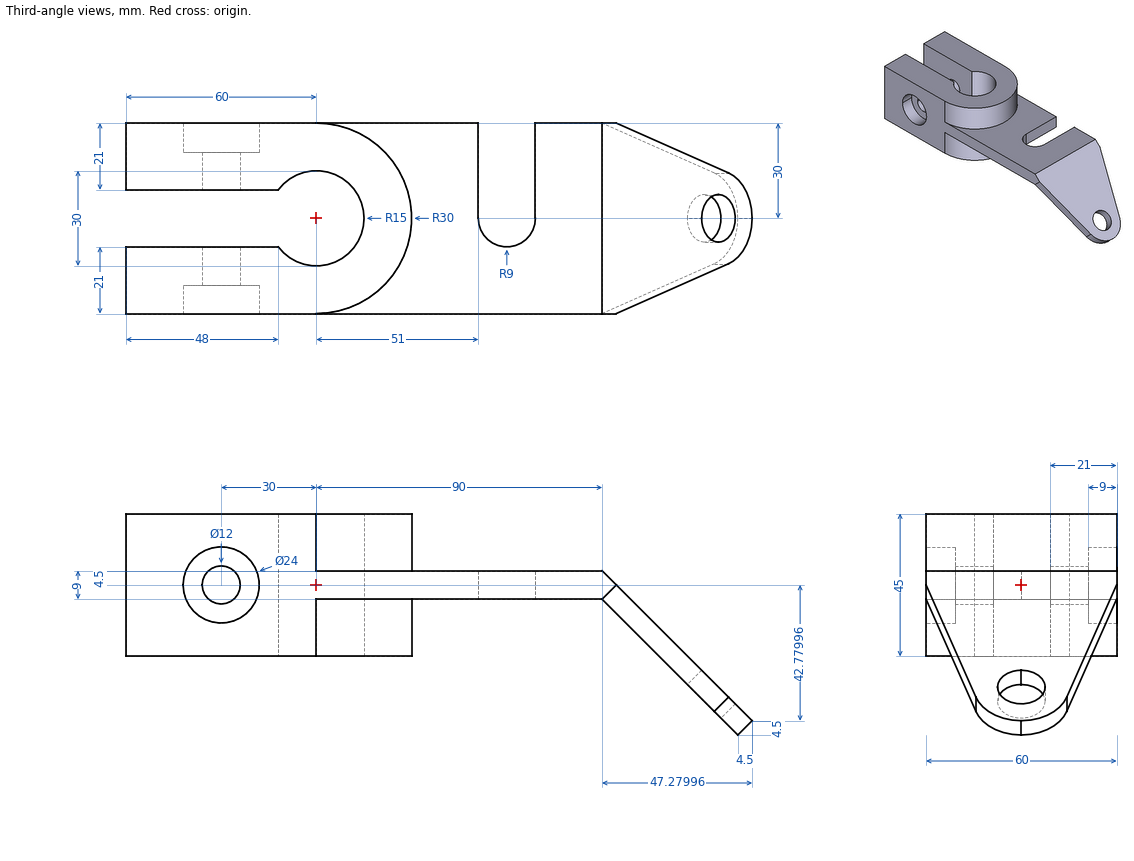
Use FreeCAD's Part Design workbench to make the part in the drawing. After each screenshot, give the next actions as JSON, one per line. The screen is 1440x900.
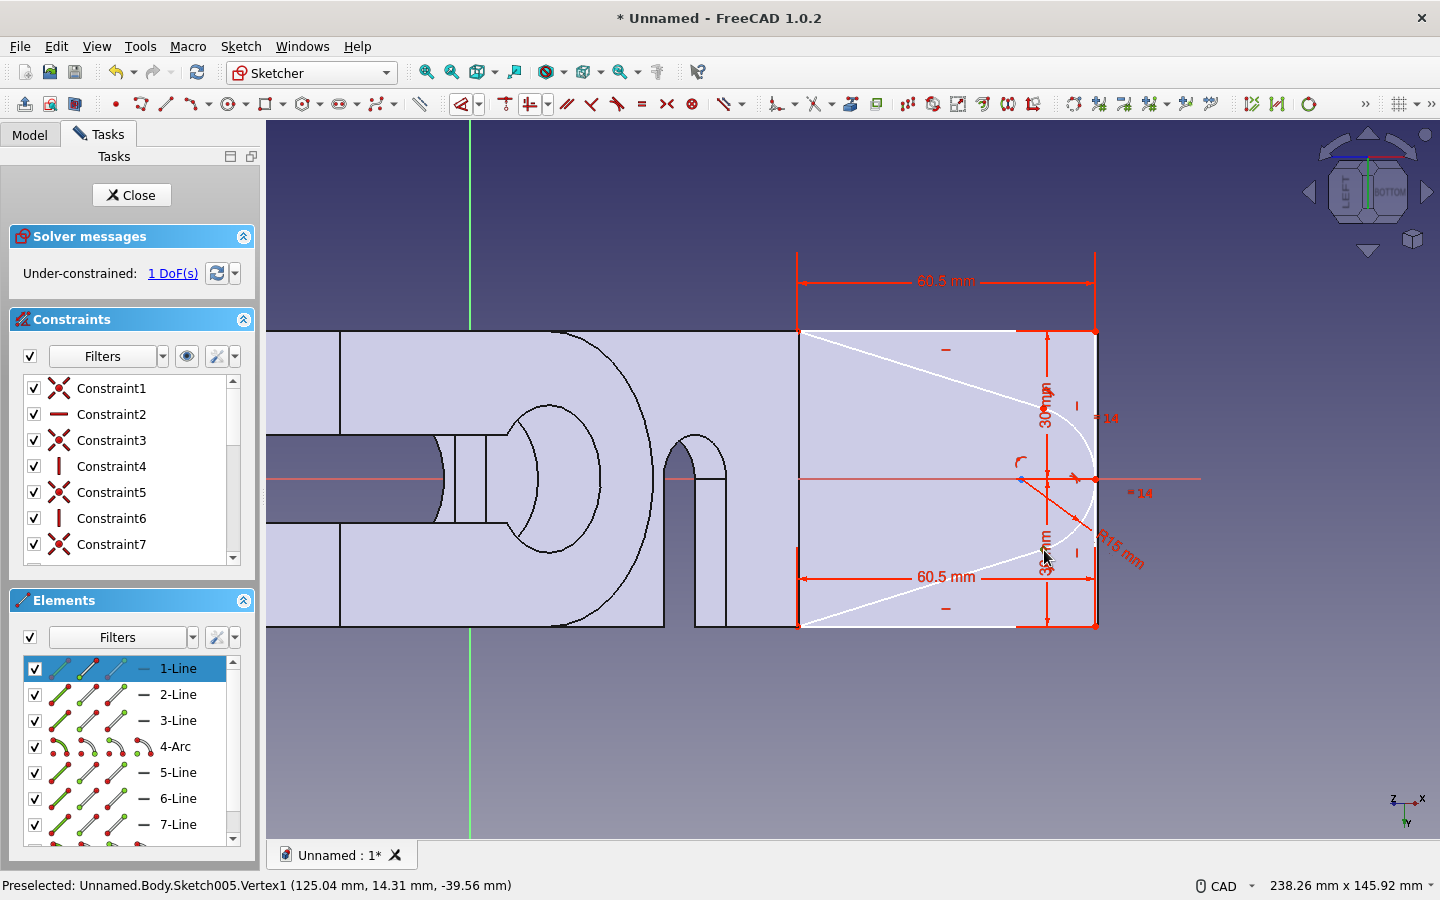
{"action": "left_click", "coordinate": [478, 104]}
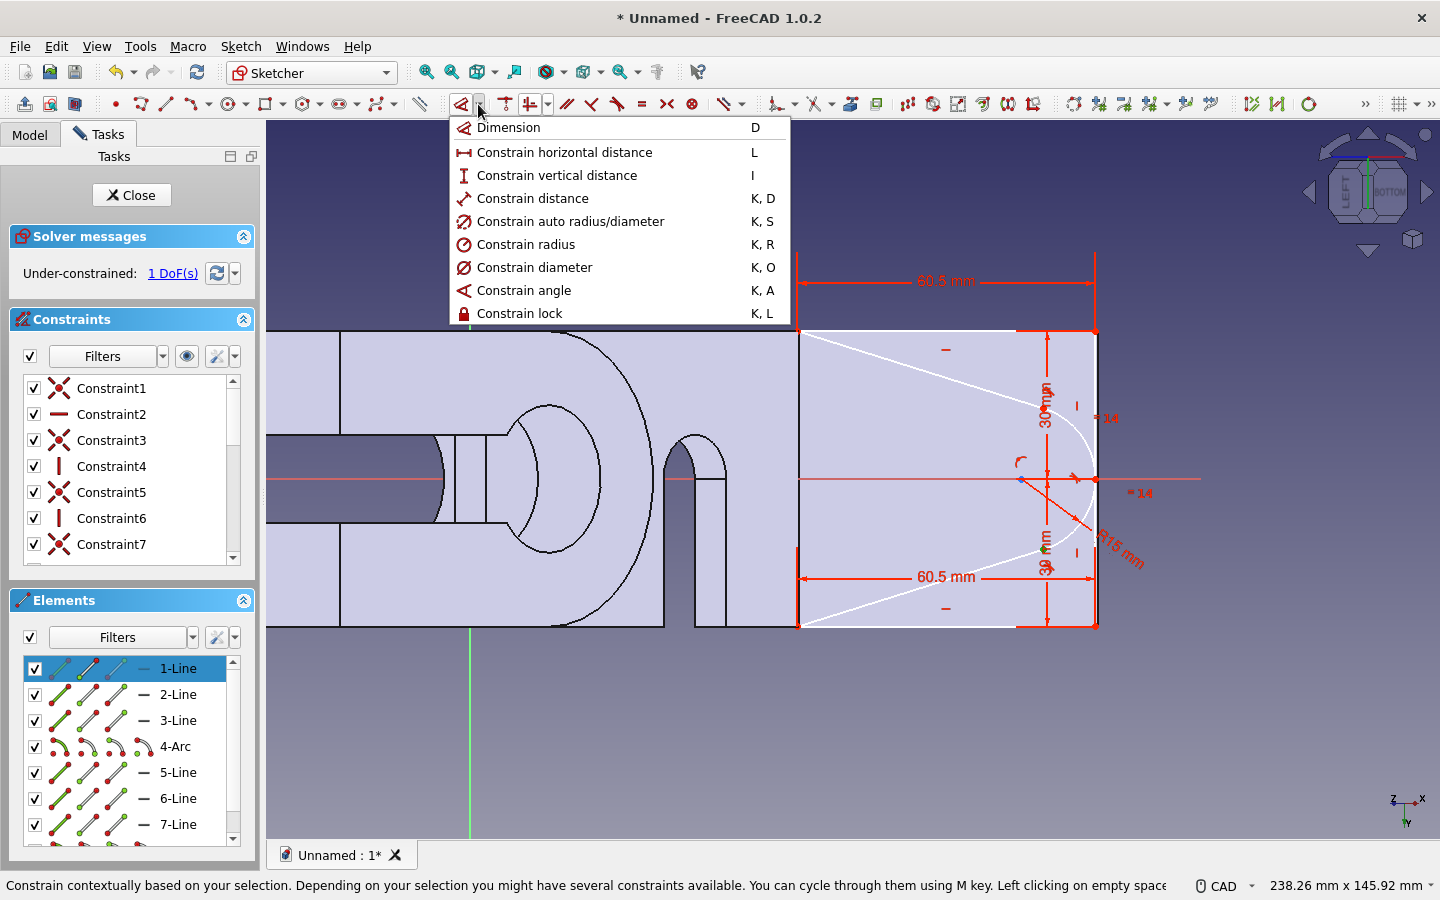
{"action": "left_click", "coordinate": [620, 152]}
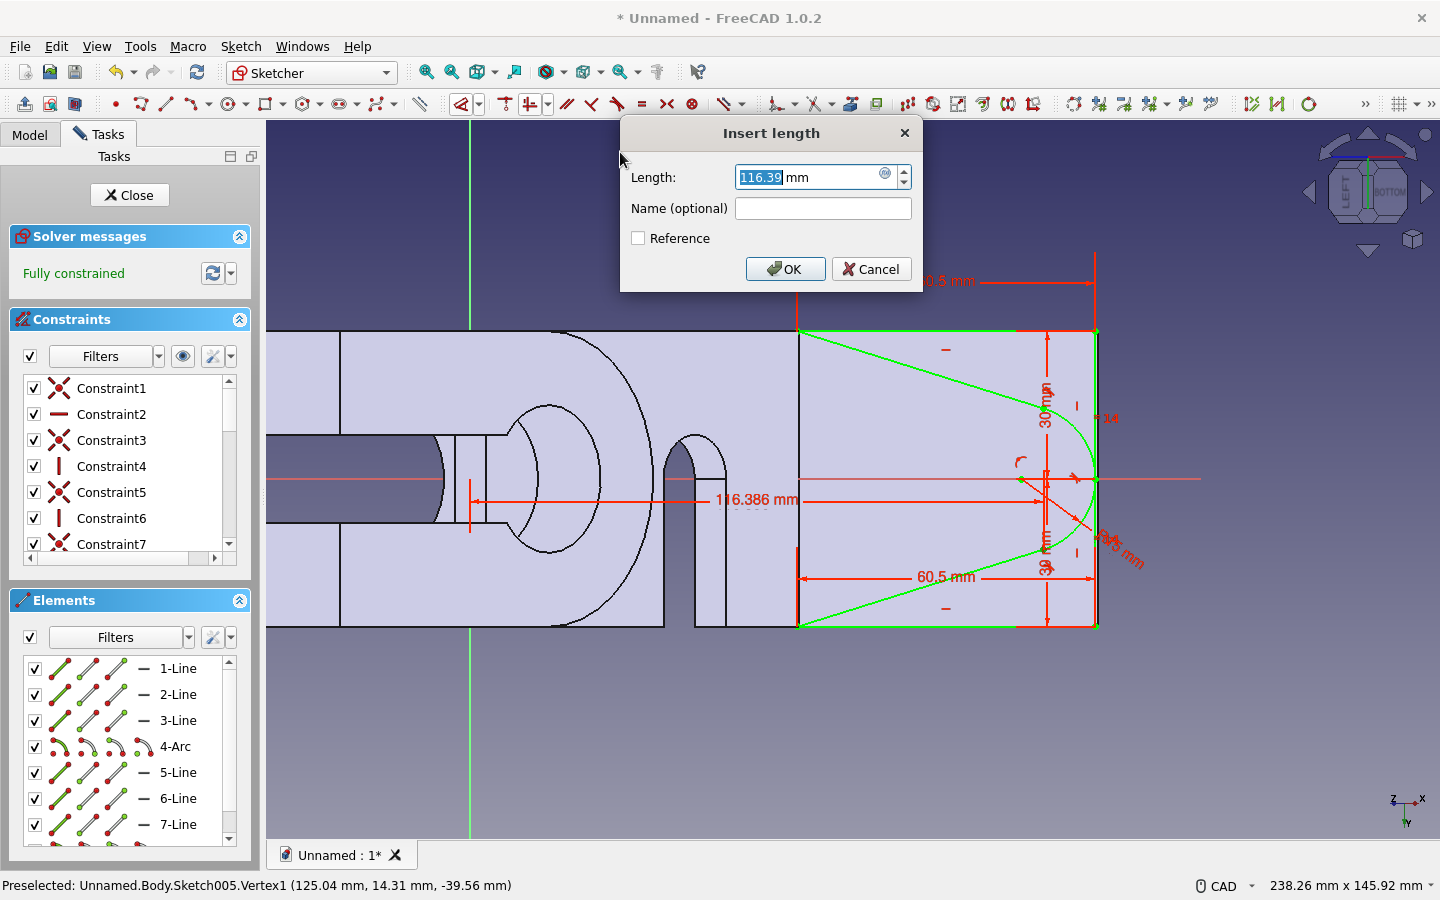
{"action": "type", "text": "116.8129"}
{"action": "key", "text": "Return"}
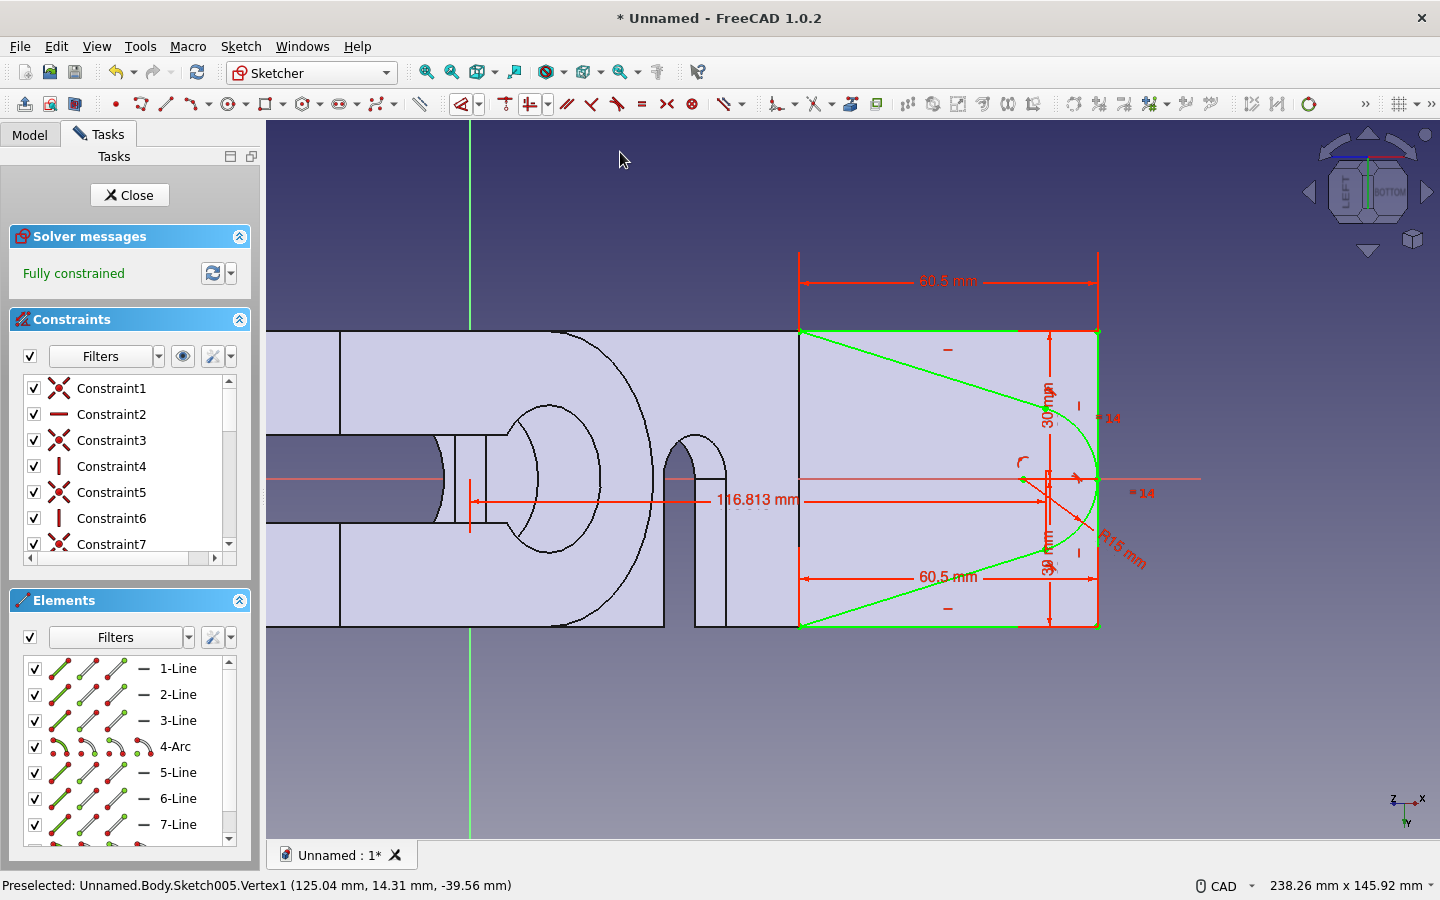
{"action": "left_click", "coordinate": [130, 195]}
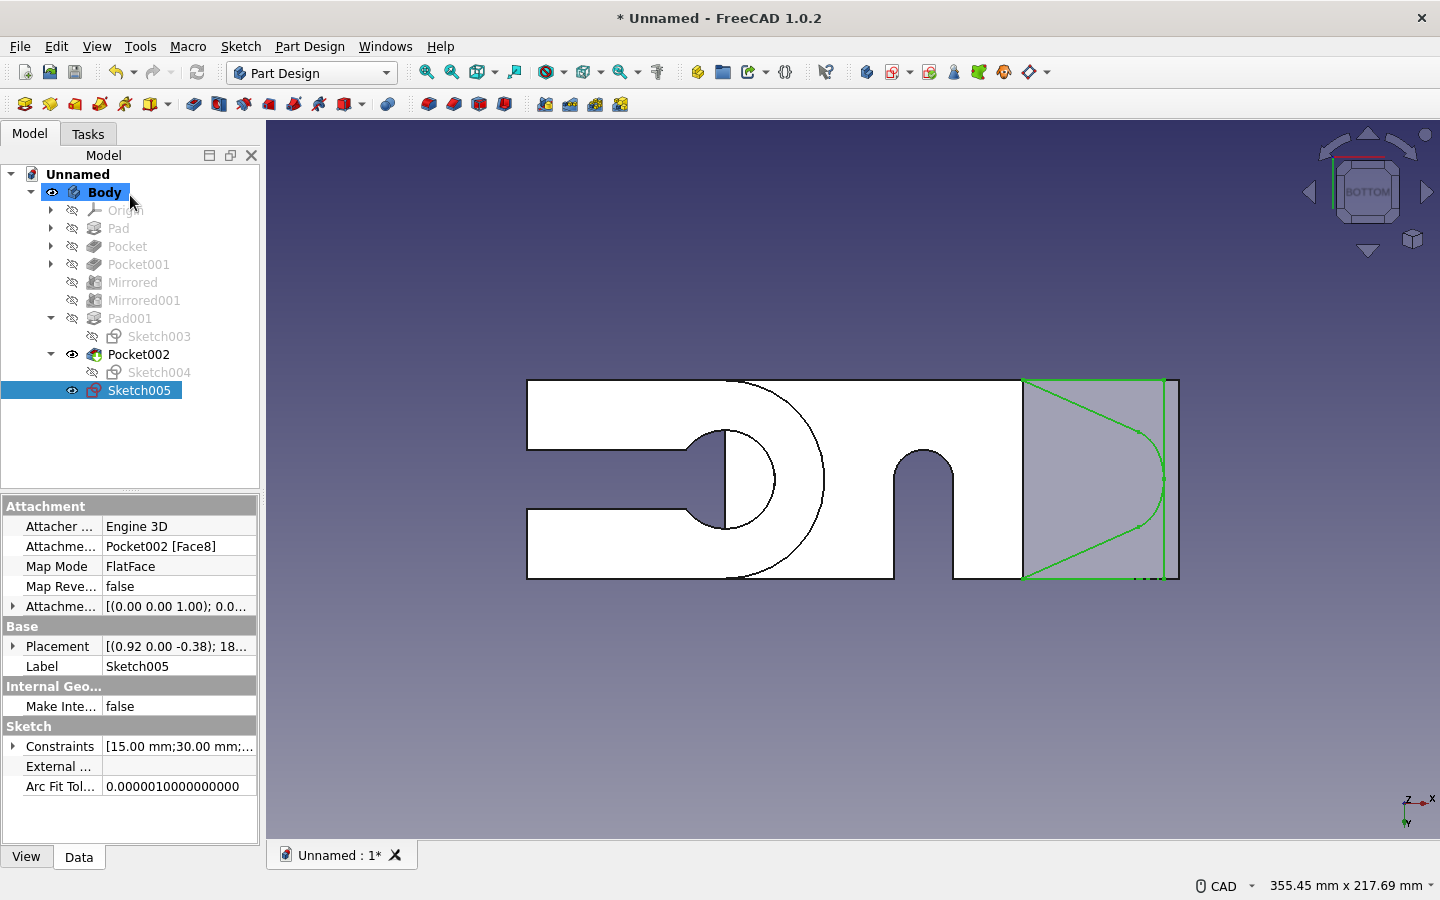
{"action": "left_click", "coordinate": [194, 104]}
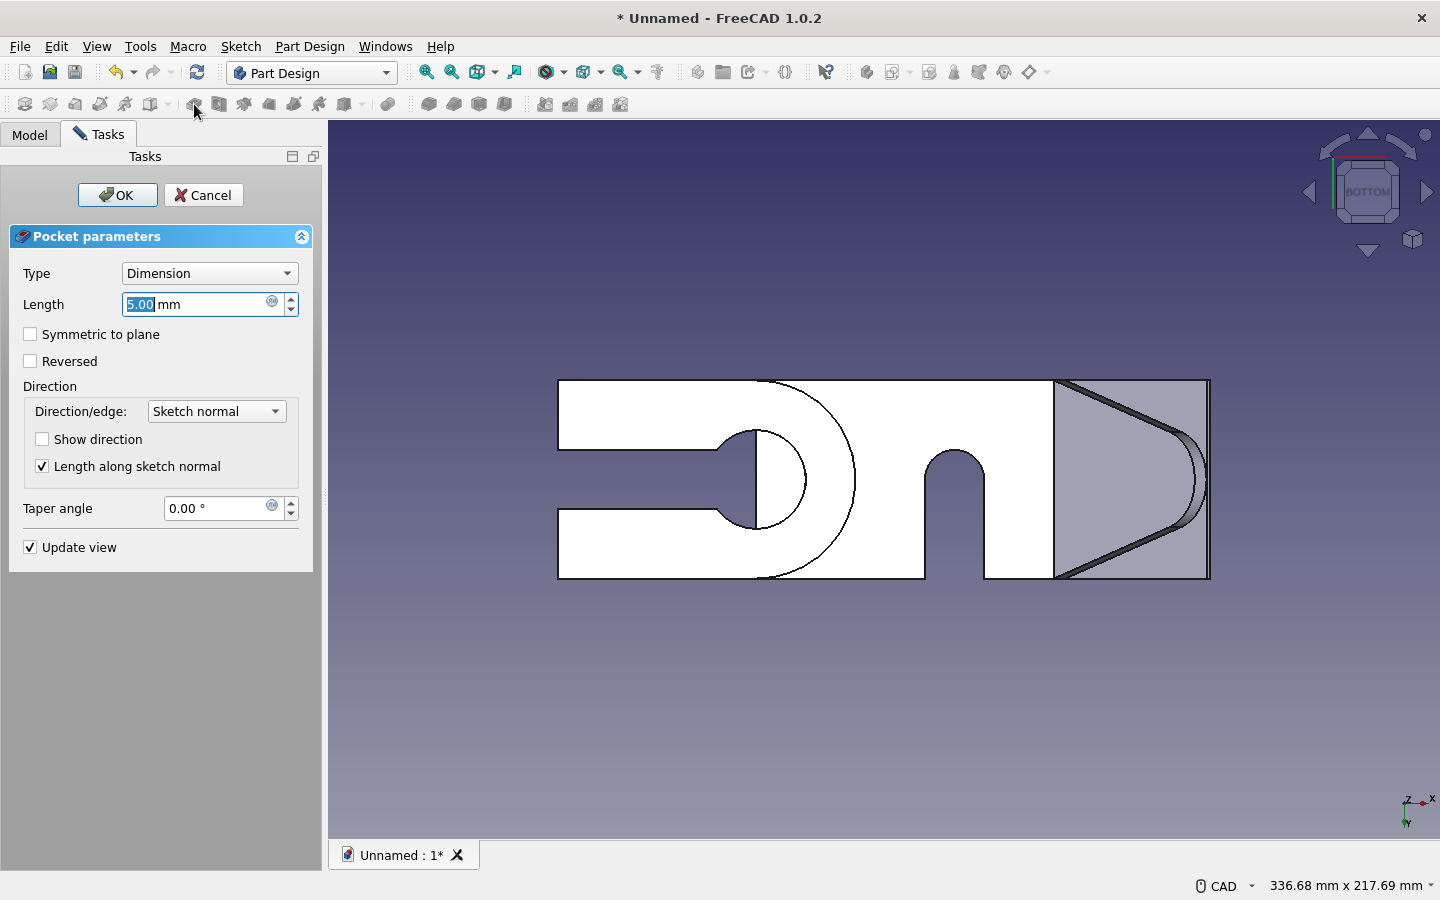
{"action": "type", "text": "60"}
{"action": "key", "text": "Tab"}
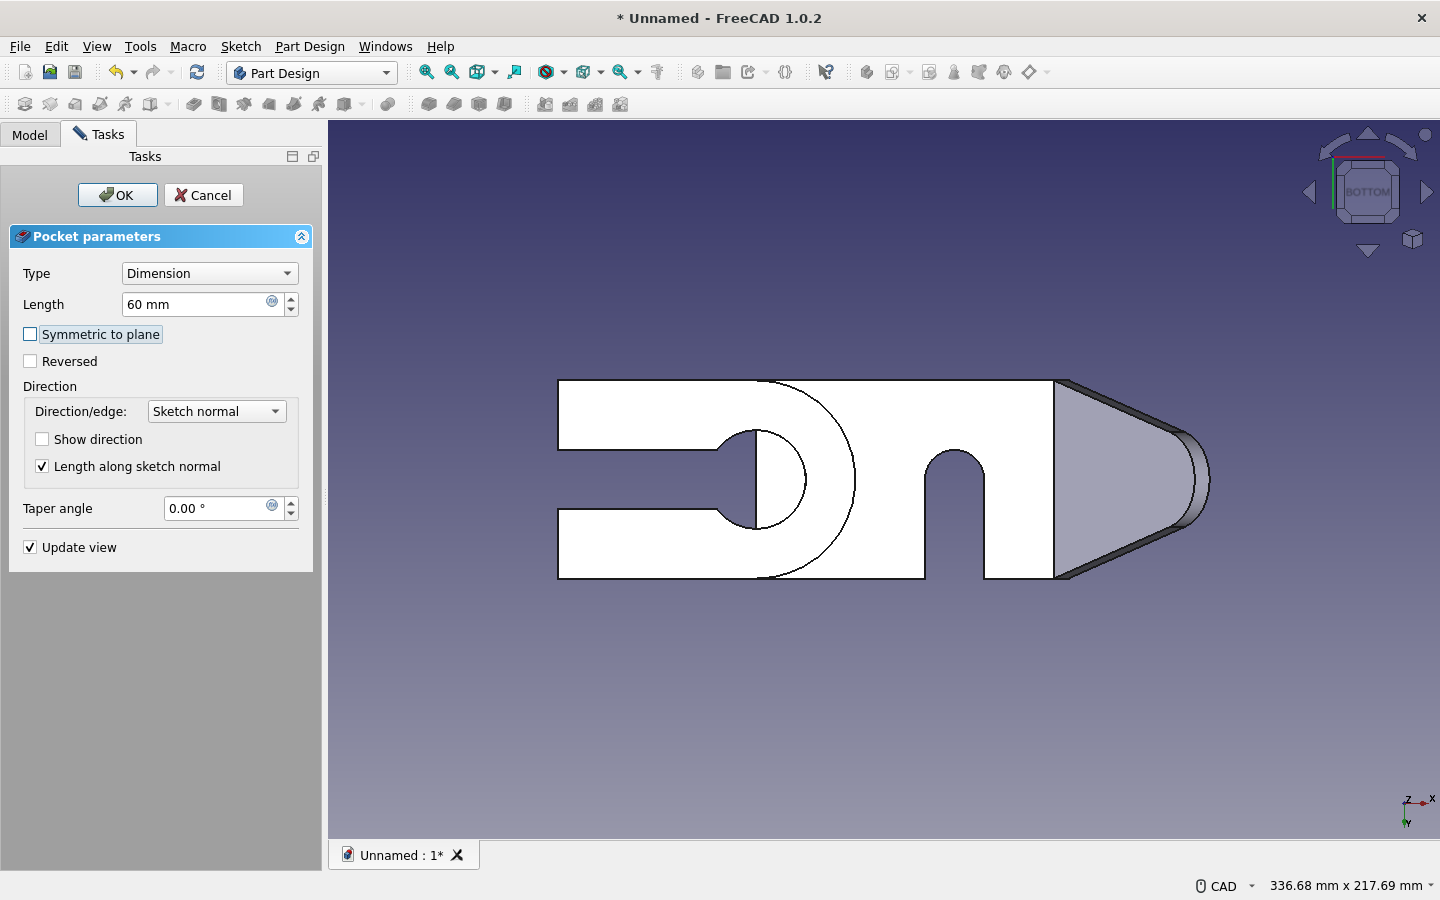
{"action": "left_click", "coordinate": [31, 334]}